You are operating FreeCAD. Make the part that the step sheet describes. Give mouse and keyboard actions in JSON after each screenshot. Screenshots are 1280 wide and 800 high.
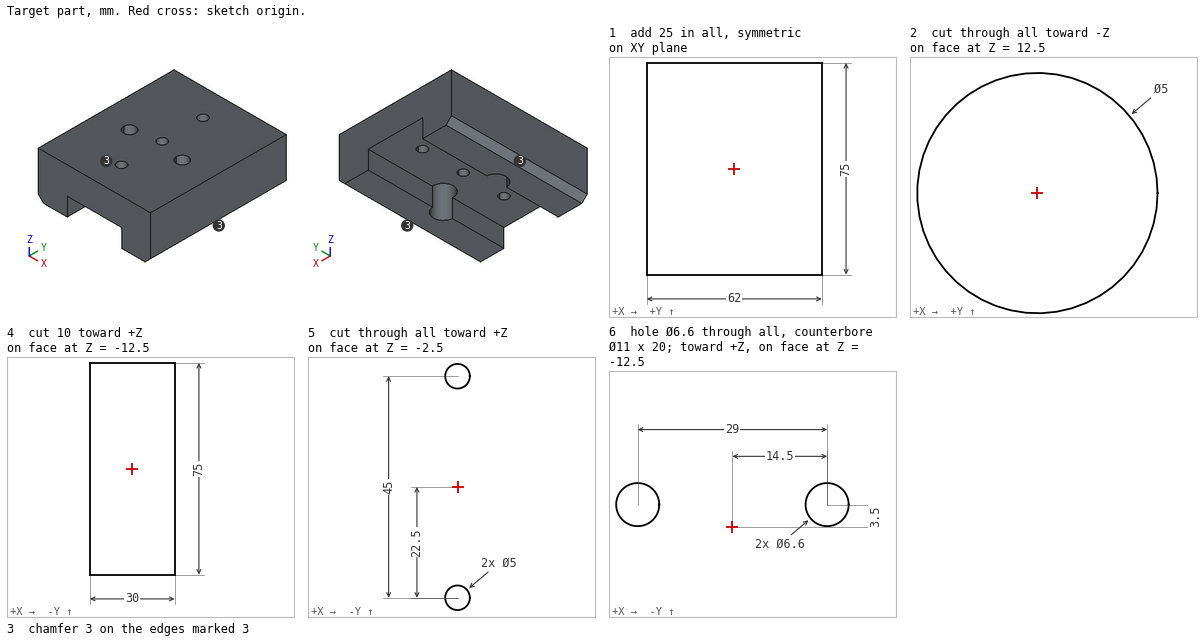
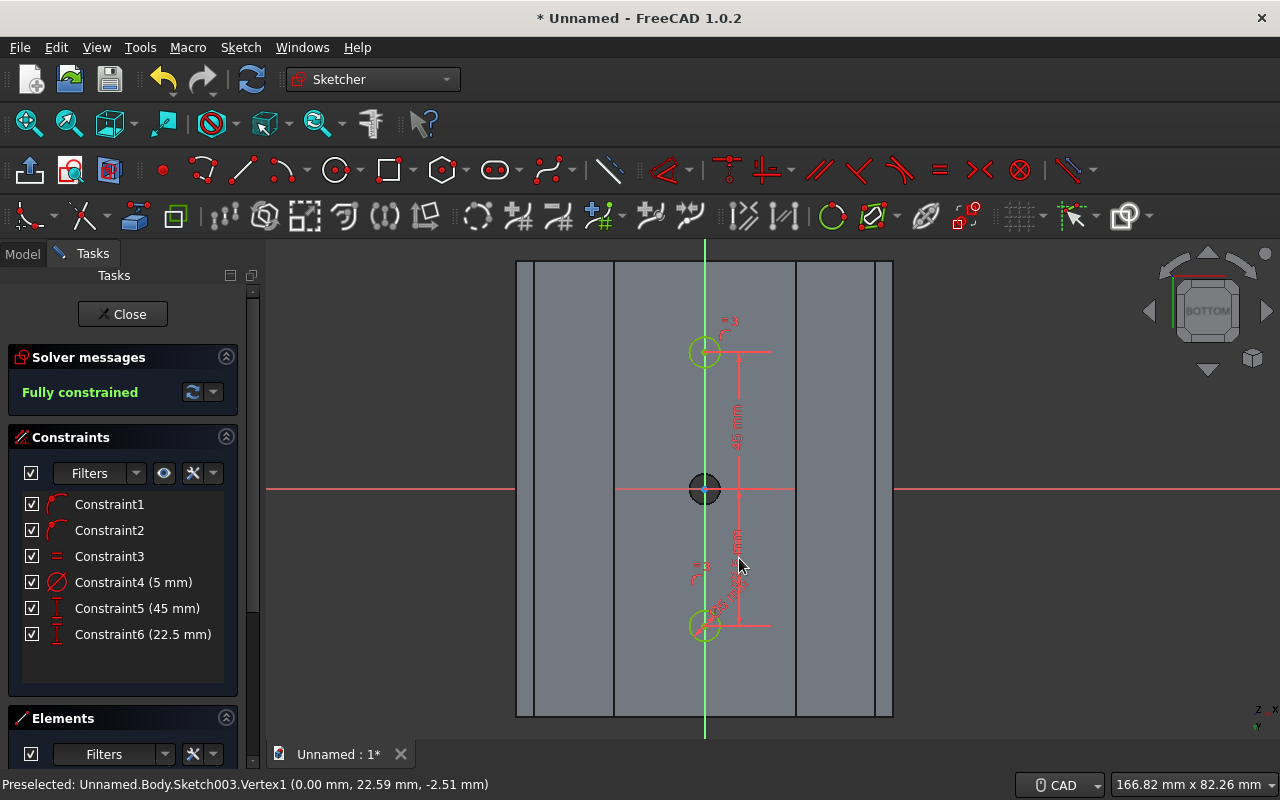
{"action": "left_click", "coordinate": [123, 314]}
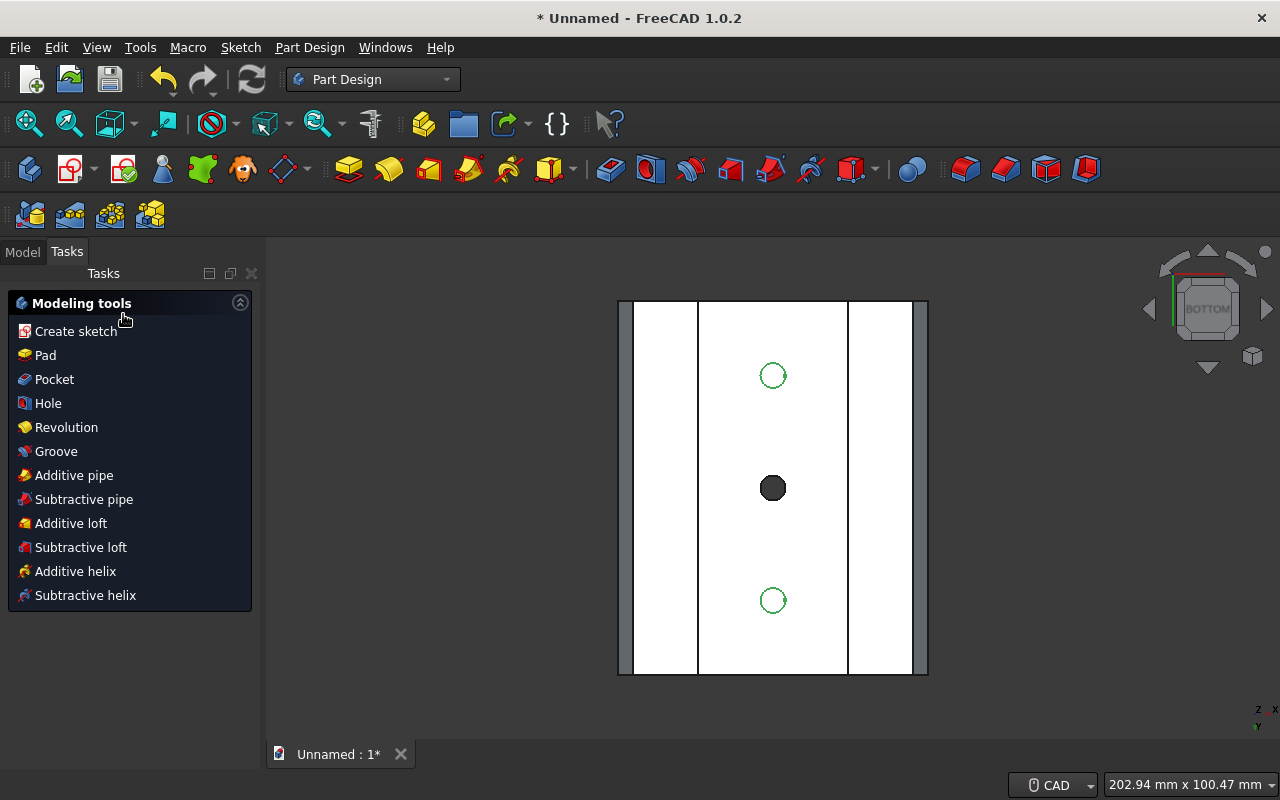
{"action": "left_click", "coordinate": [612, 170]}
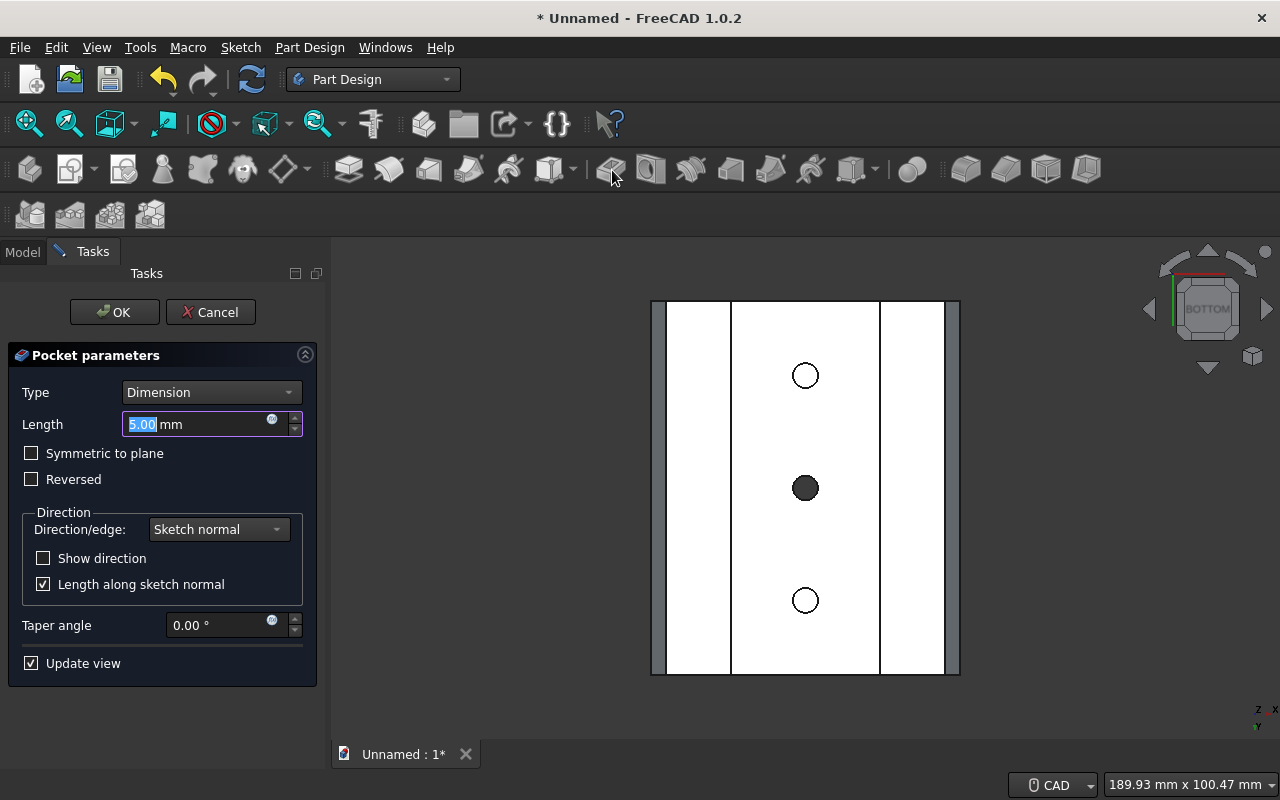
{"action": "left_click", "coordinate": [212, 392]}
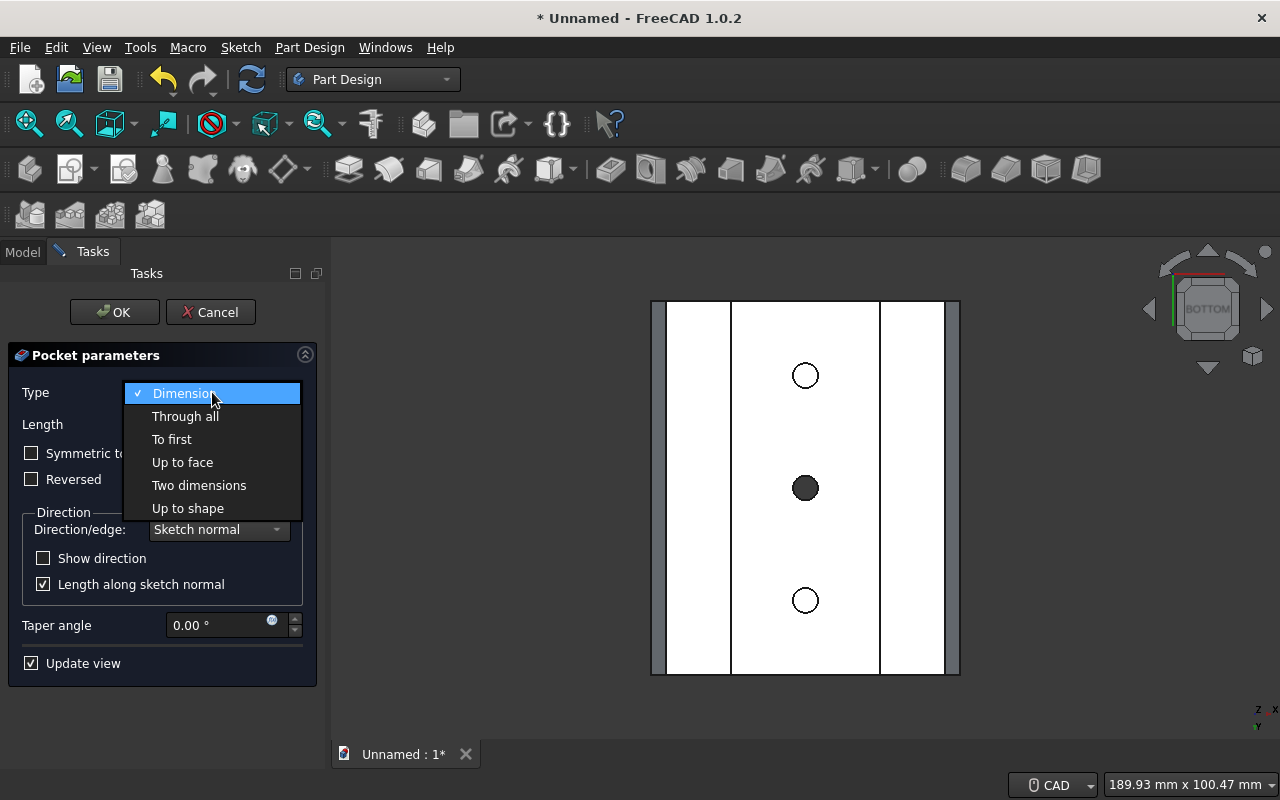
{"action": "left_click", "coordinate": [212, 416]}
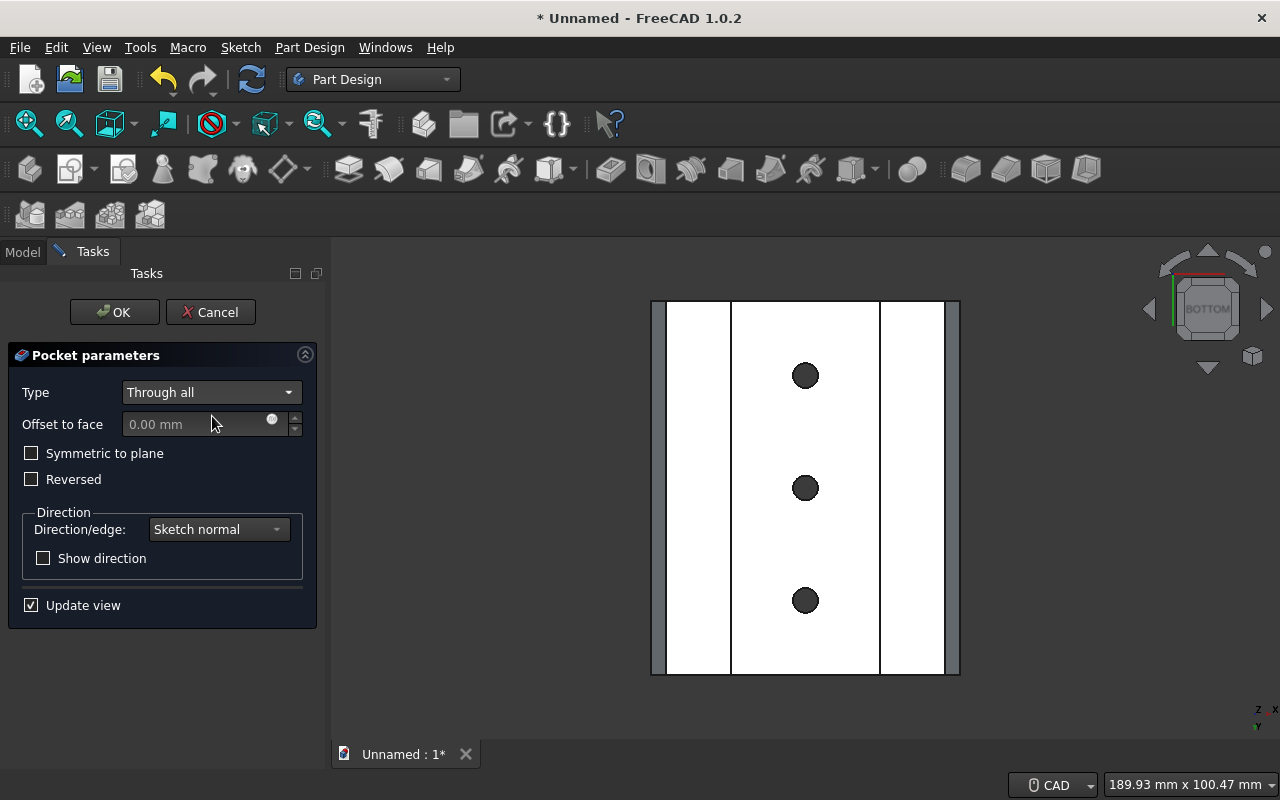
{"action": "left_click", "coordinate": [115, 312]}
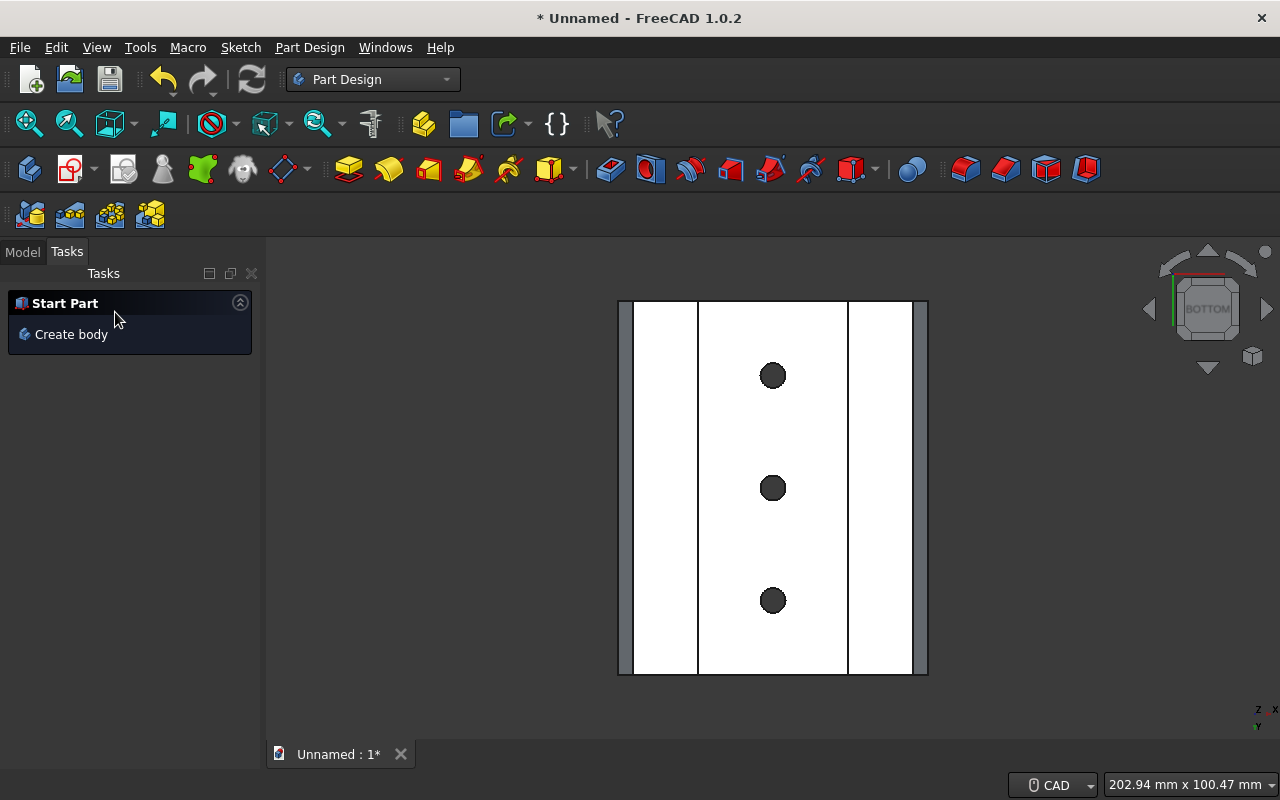
{"action": "left_click", "coordinate": [880, 594]}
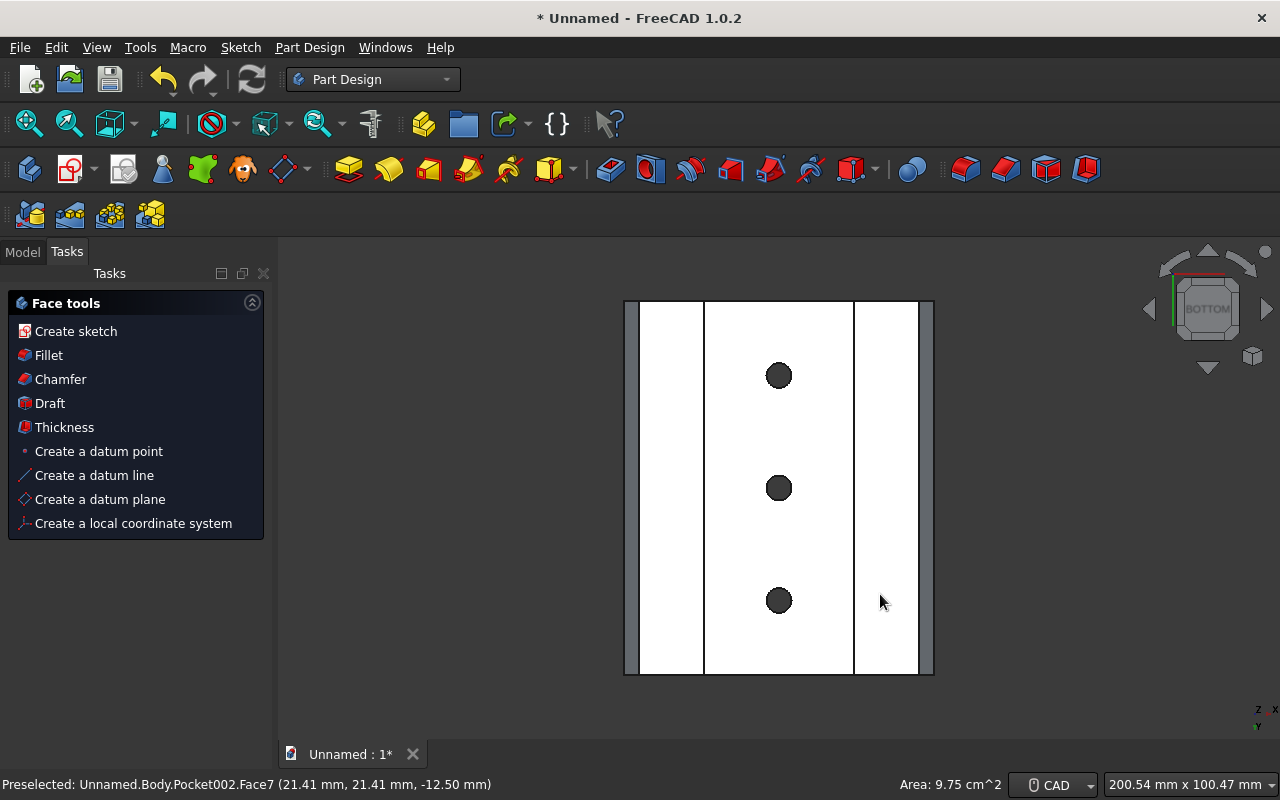
{"action": "left_click", "coordinate": [70, 170]}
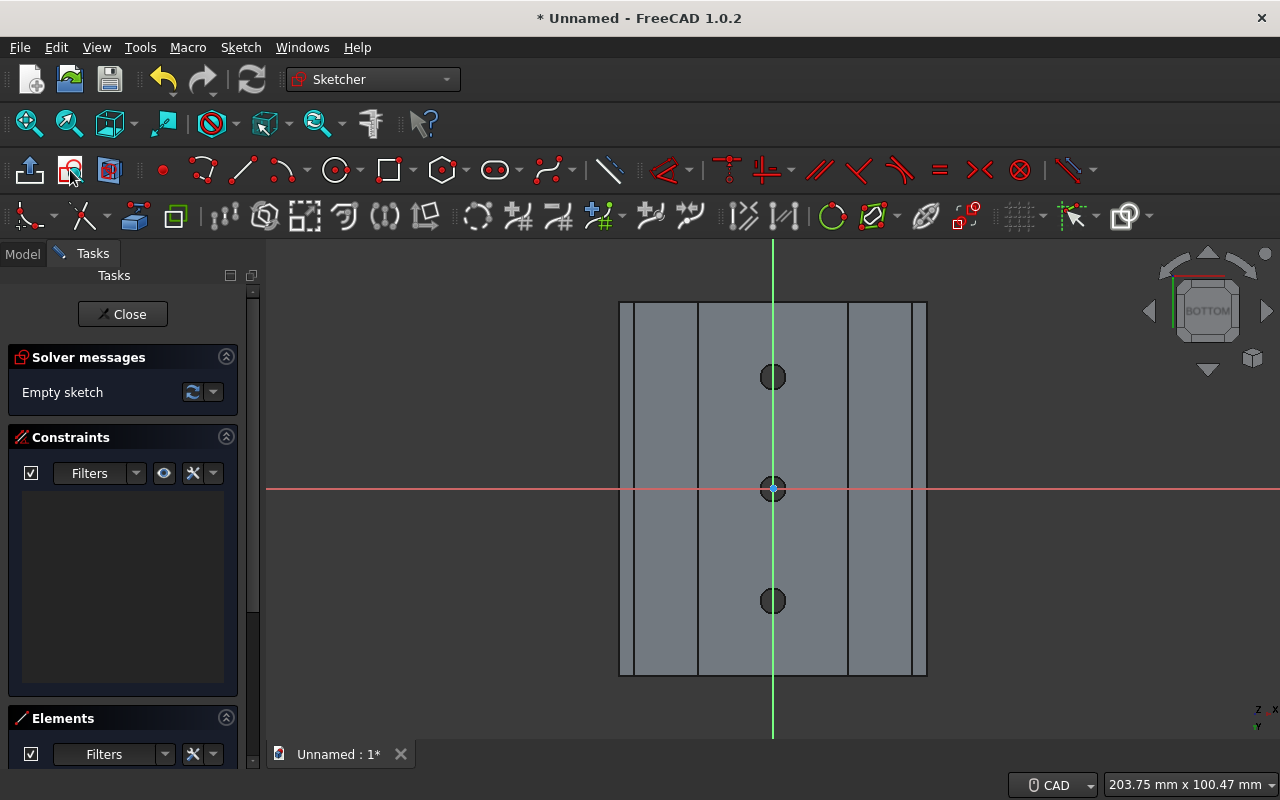
{"action": "scroll", "coordinate": [803, 465], "scroll_direction": "up", "scroll_amount": 6}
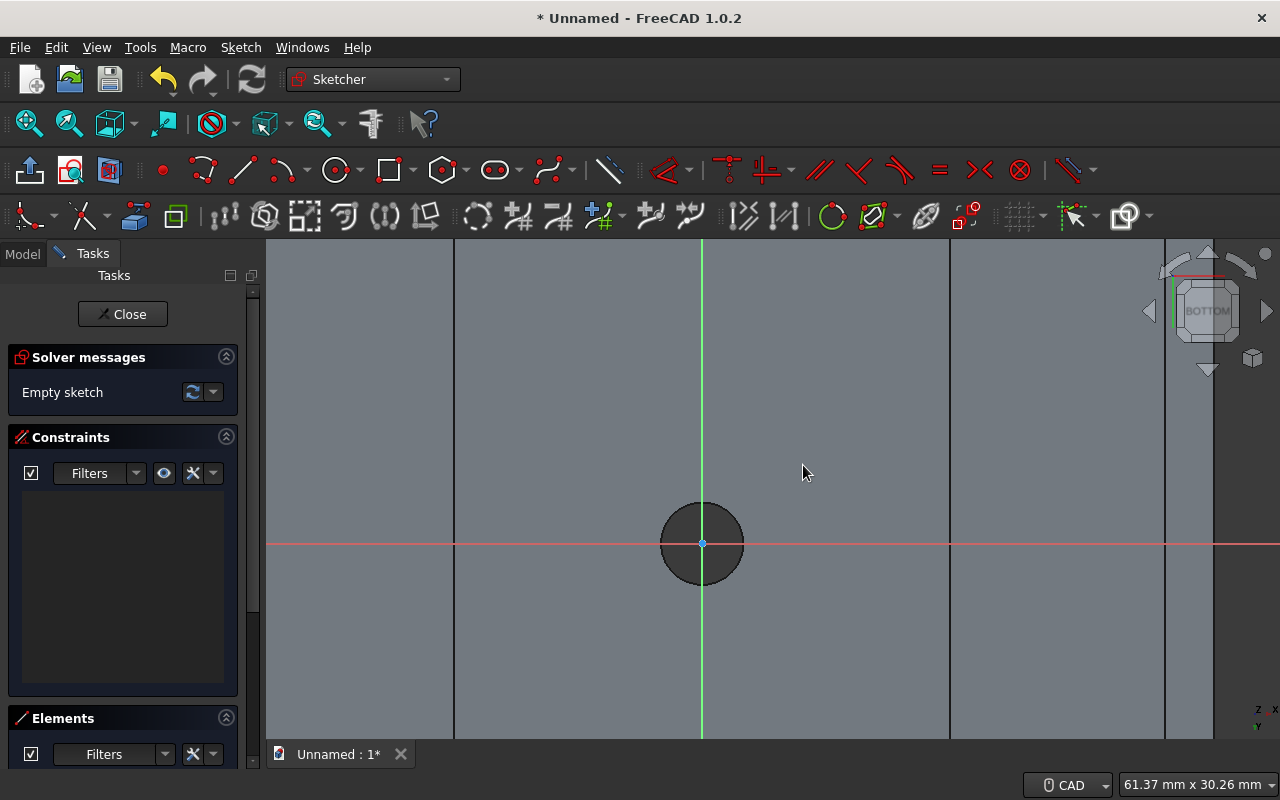
{"action": "left_click", "coordinate": [336, 170]}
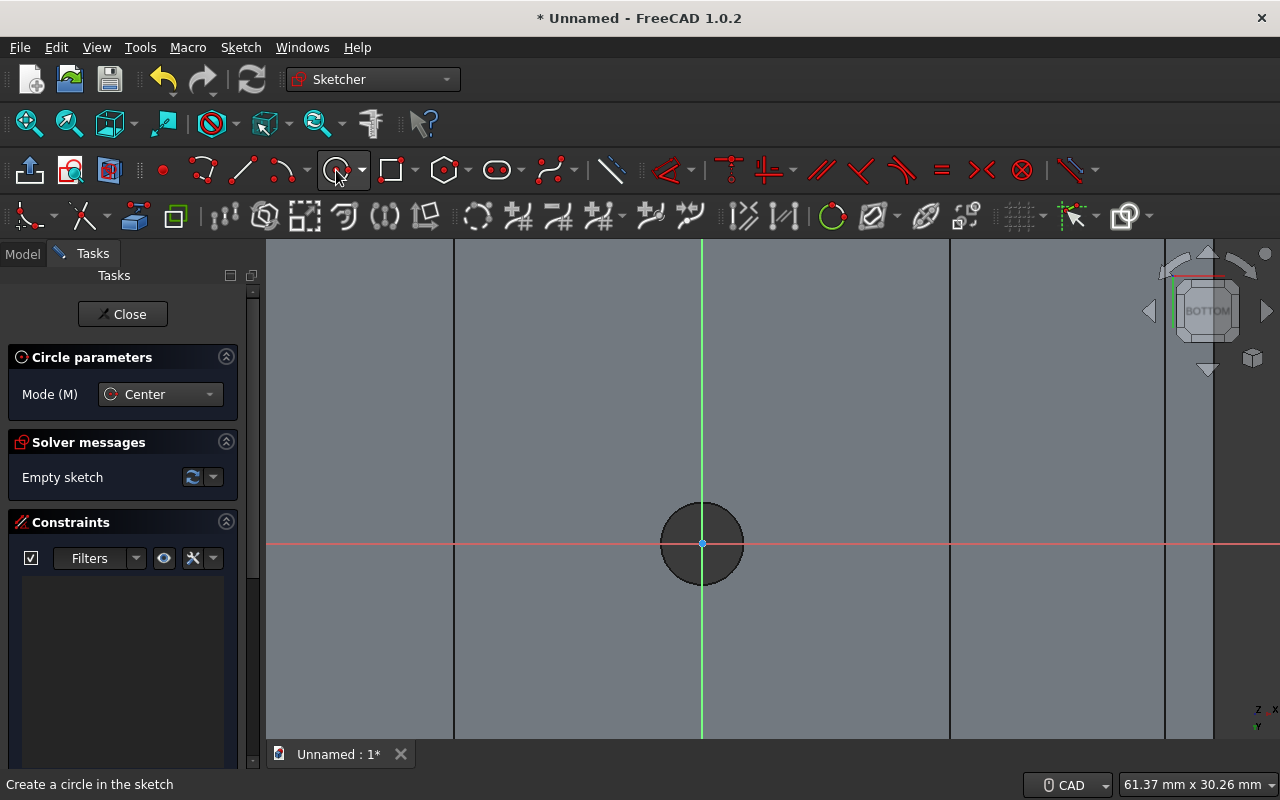
{"action": "left_click", "coordinate": [942, 486]}
{"action": "left_click", "coordinate": [980, 447]}